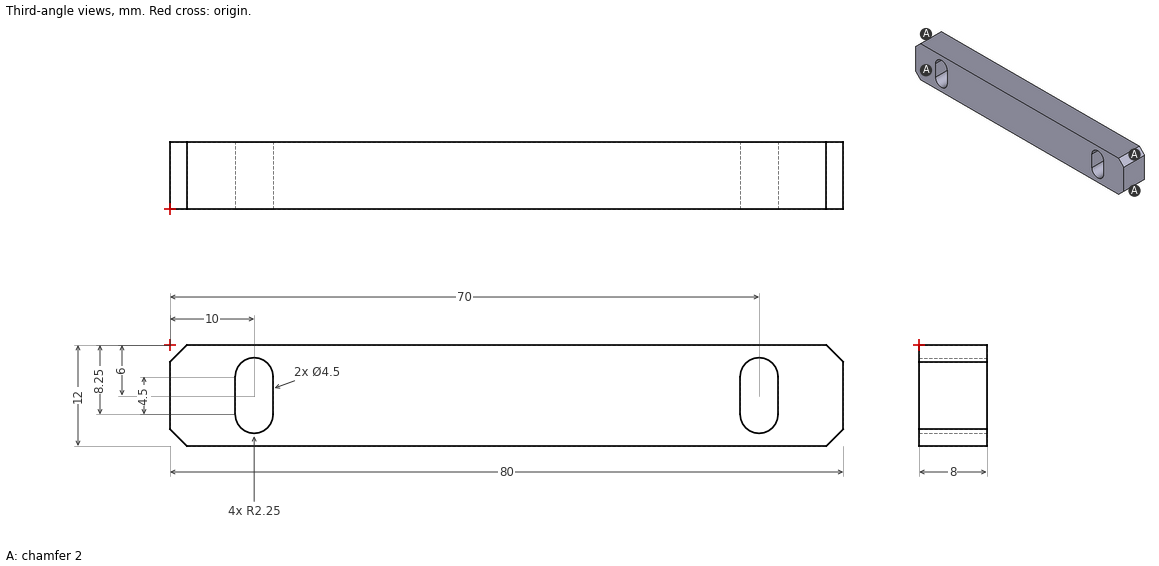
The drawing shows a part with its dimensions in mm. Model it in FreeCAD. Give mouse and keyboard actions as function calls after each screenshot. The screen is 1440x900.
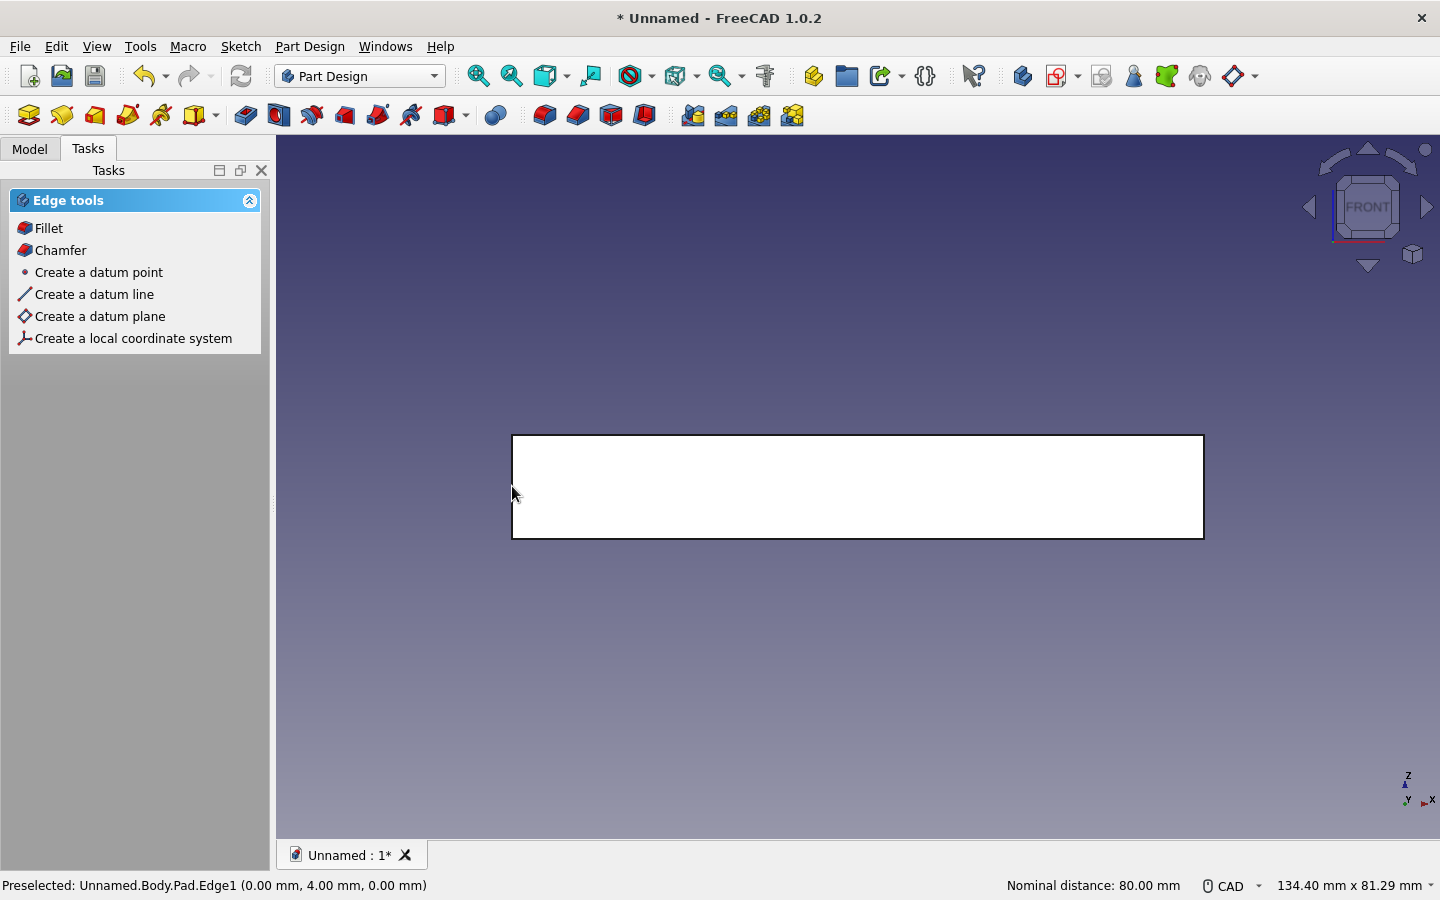
key(3)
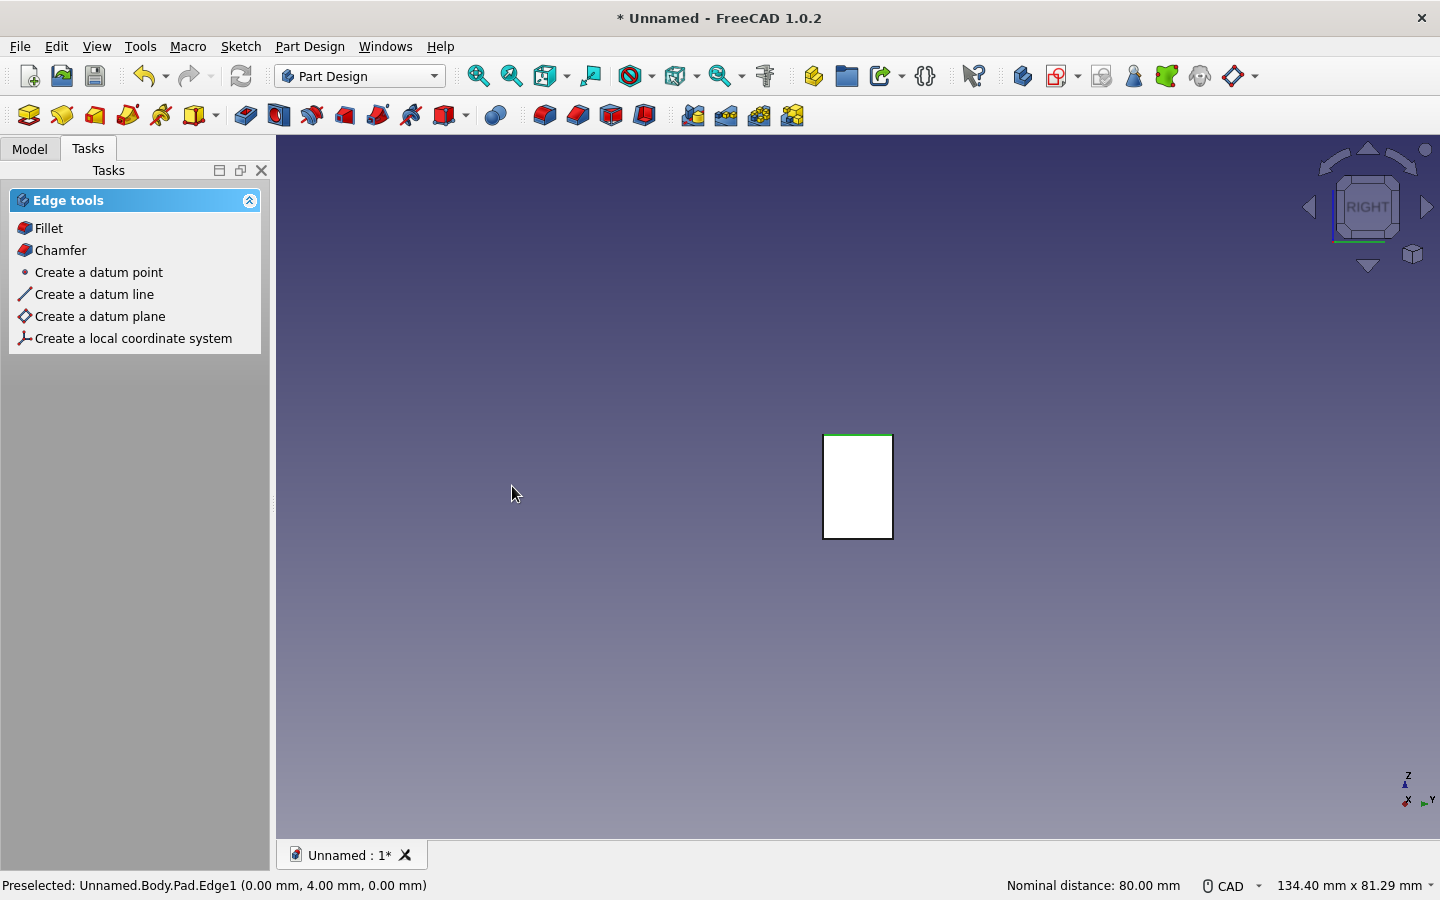
click(479, 76)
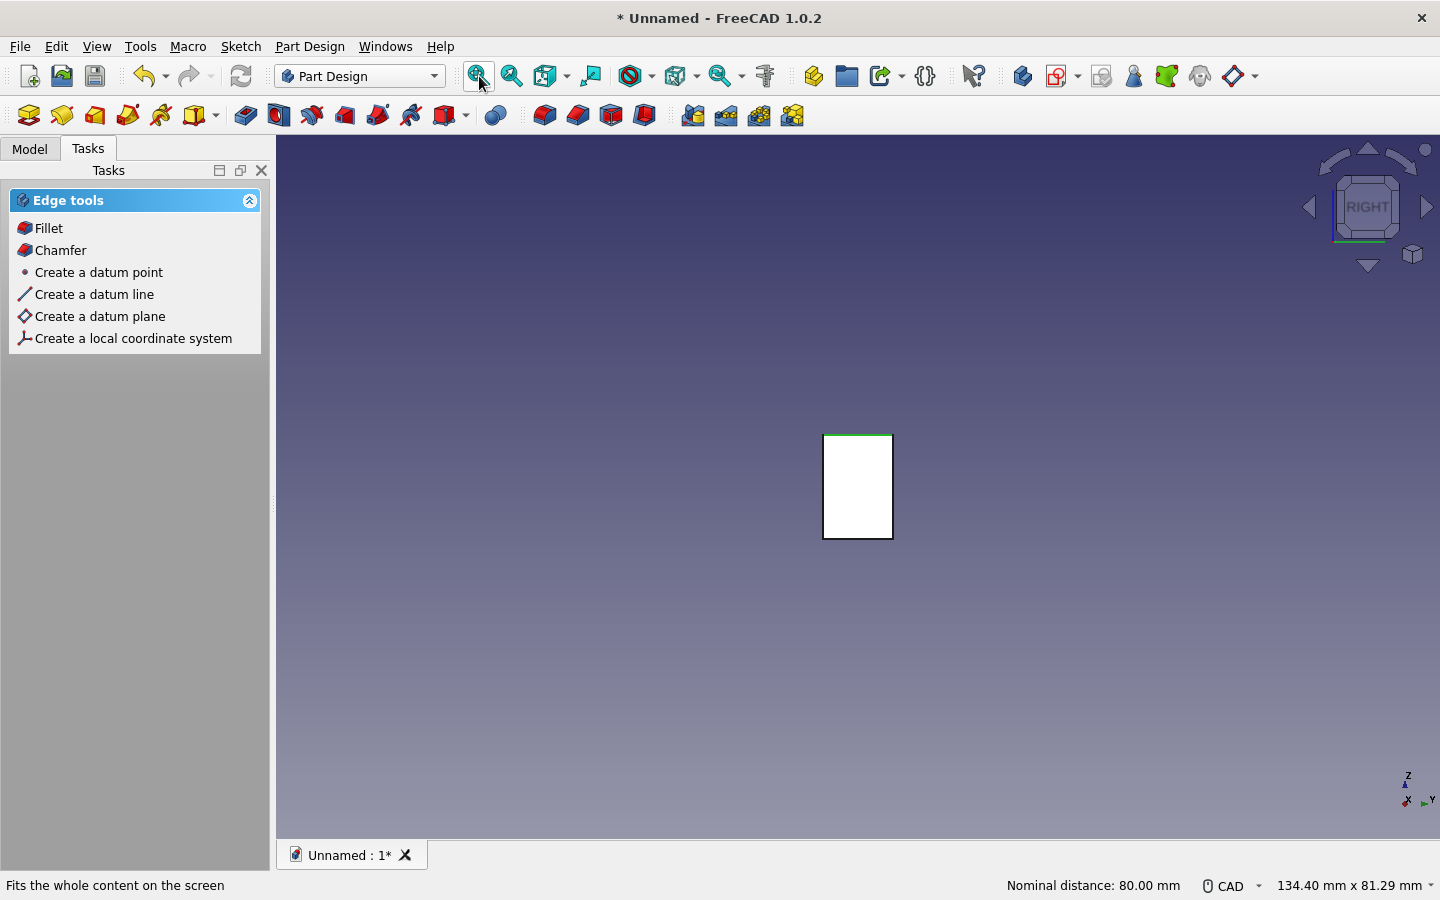
click(858, 538, ctrl)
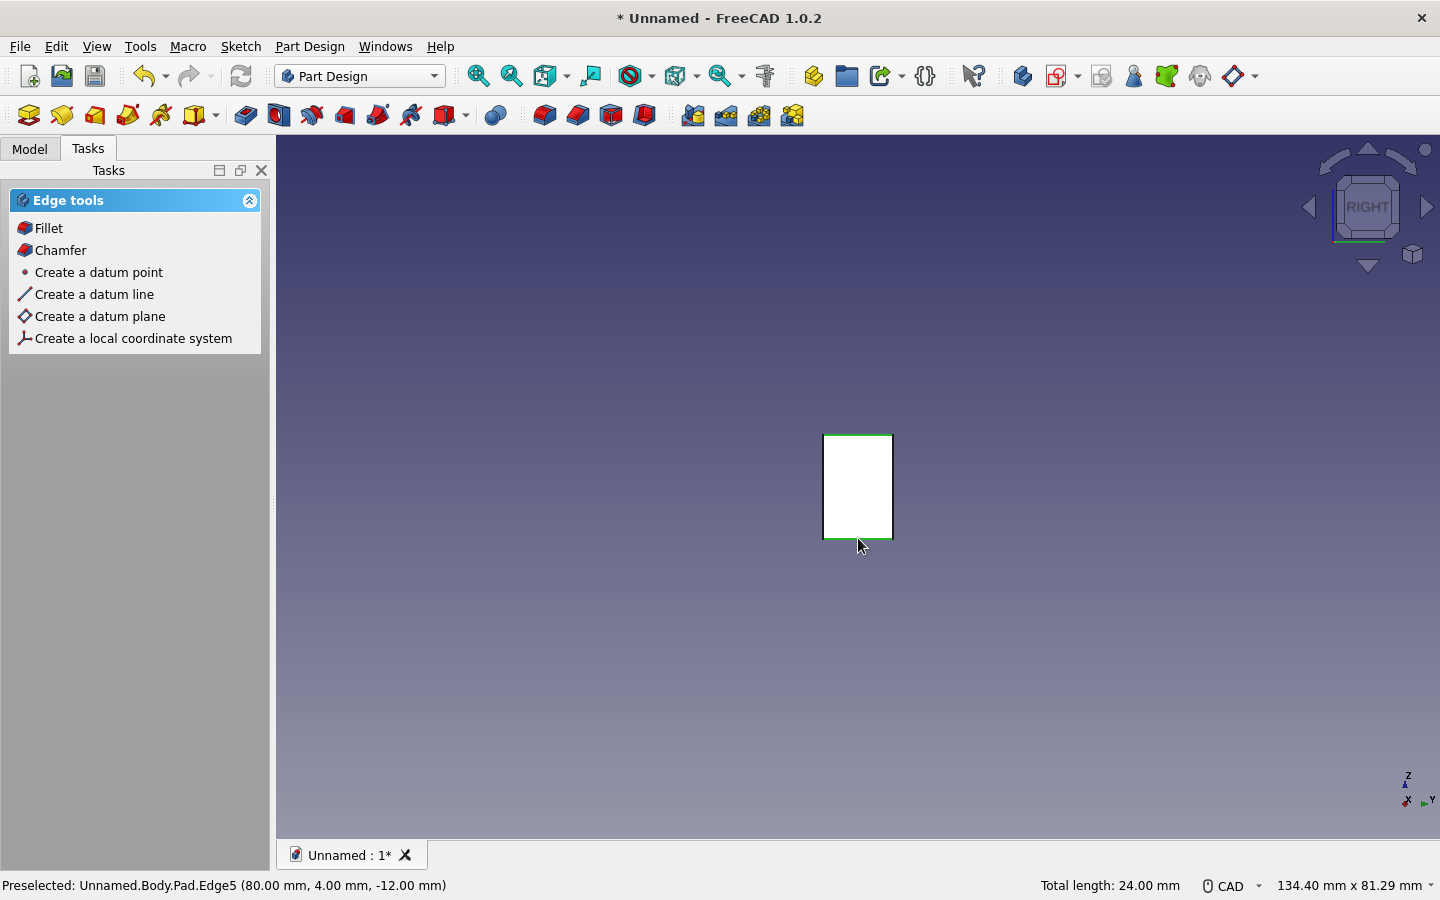
key(5)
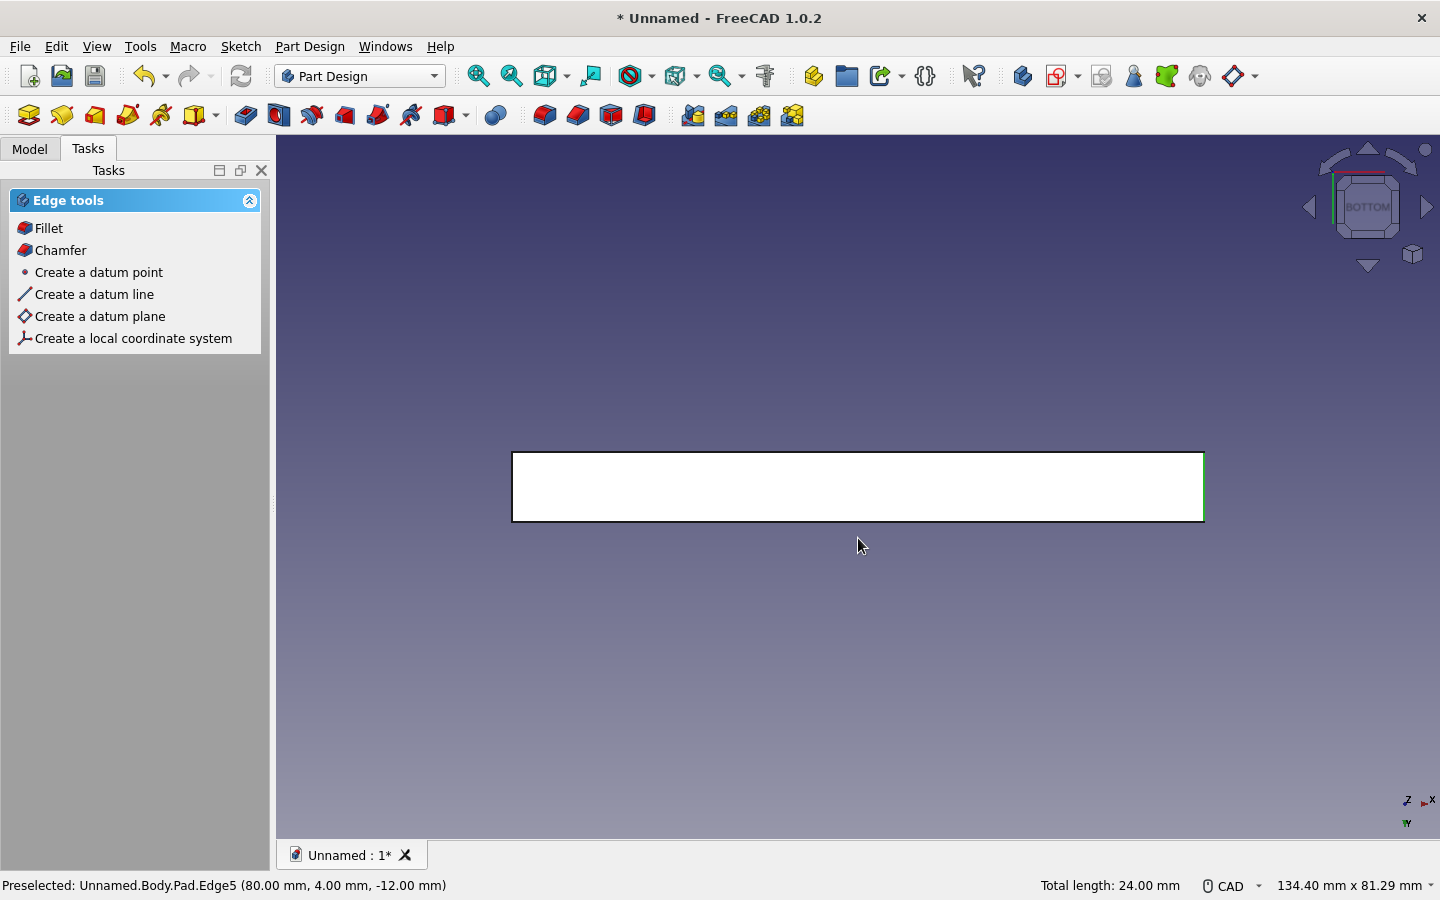
click(512, 486, ctrl)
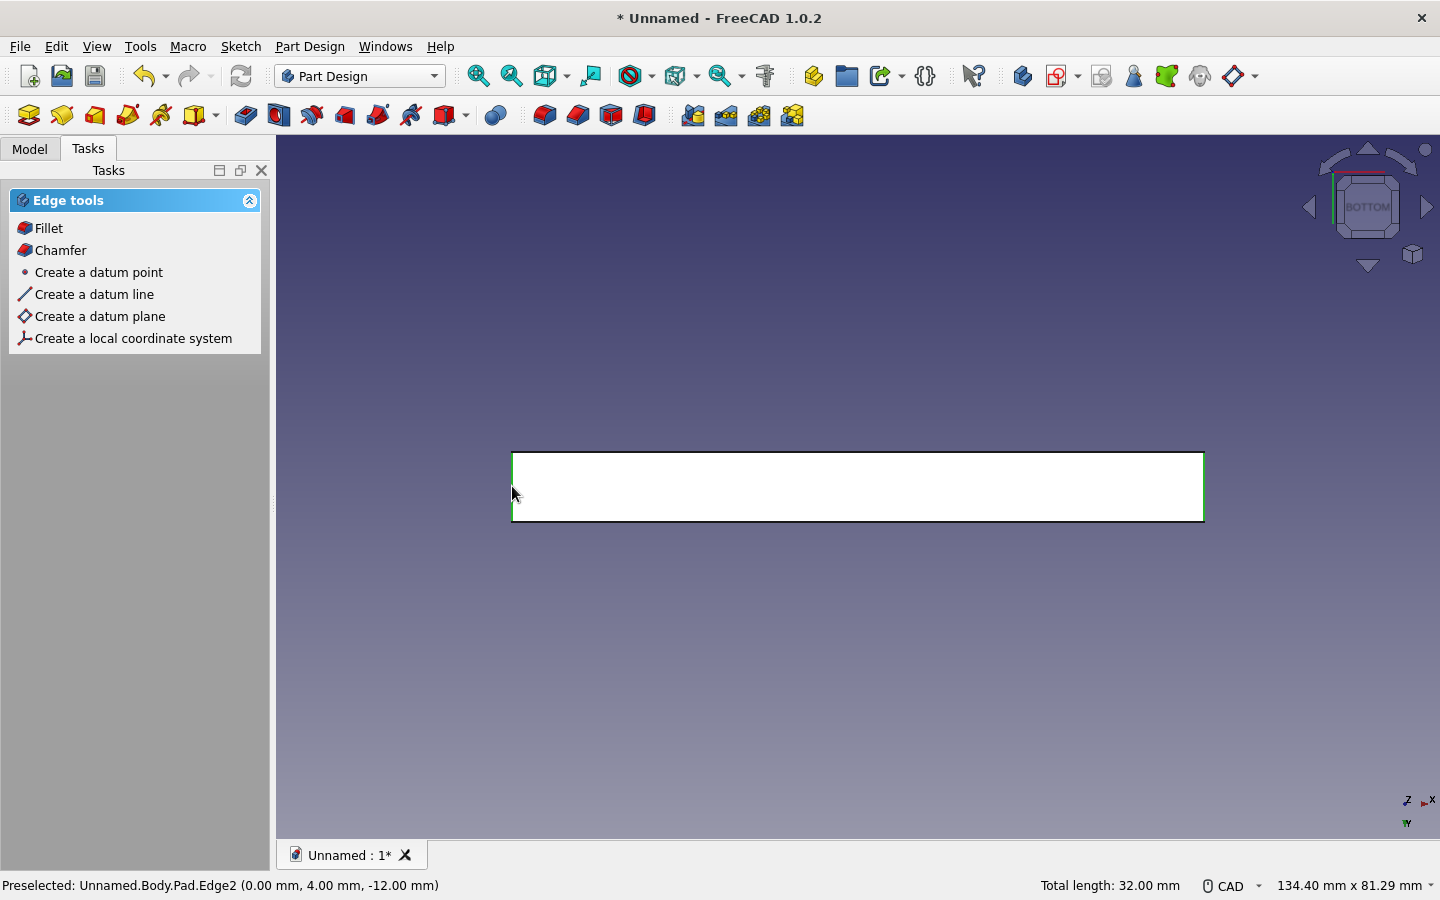
click(578, 116)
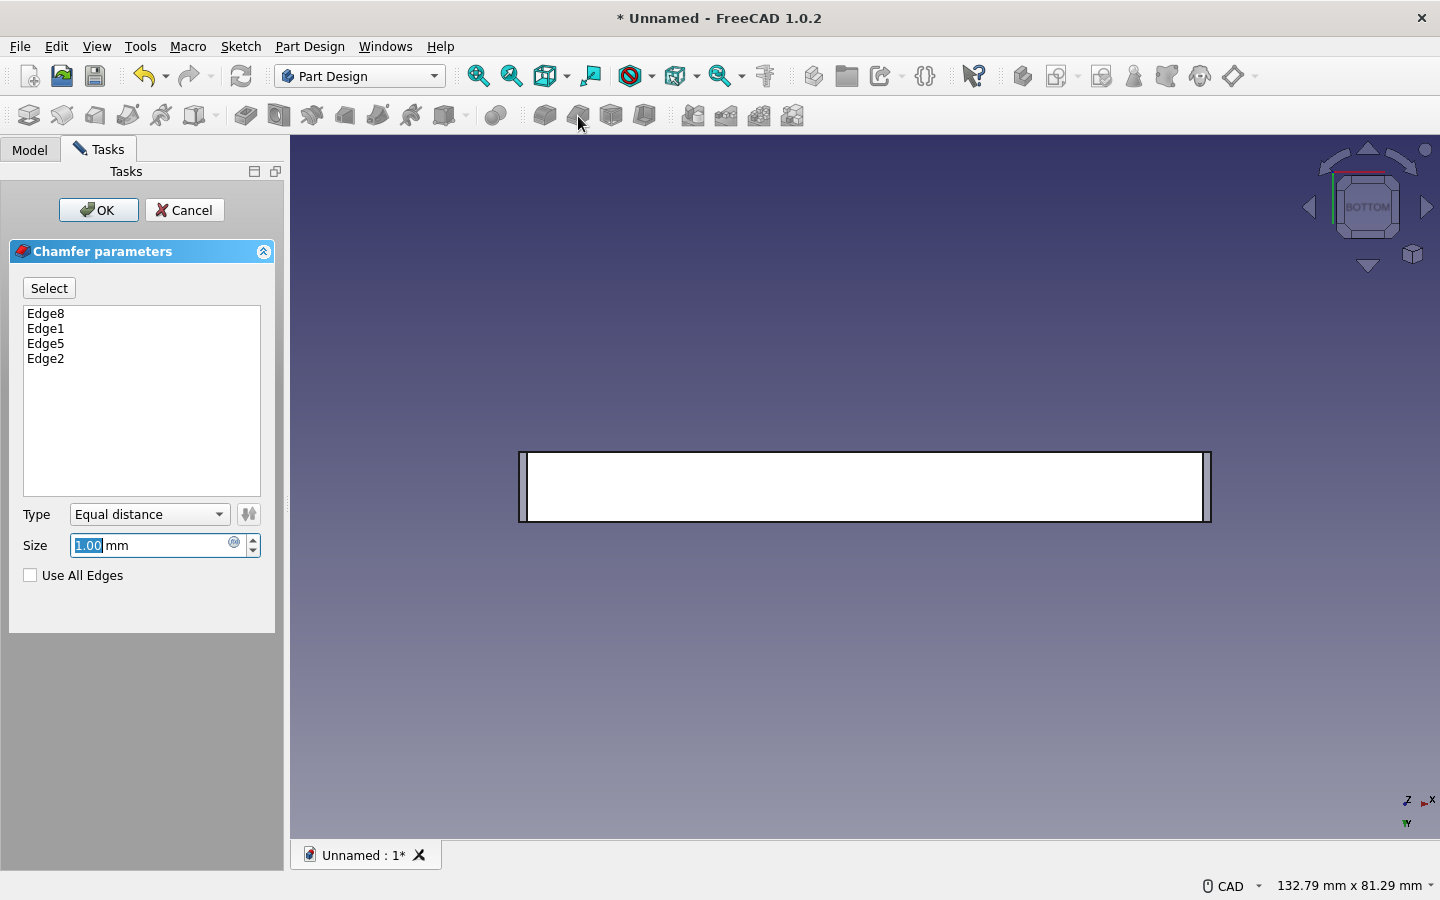
text(2)
key(Tab)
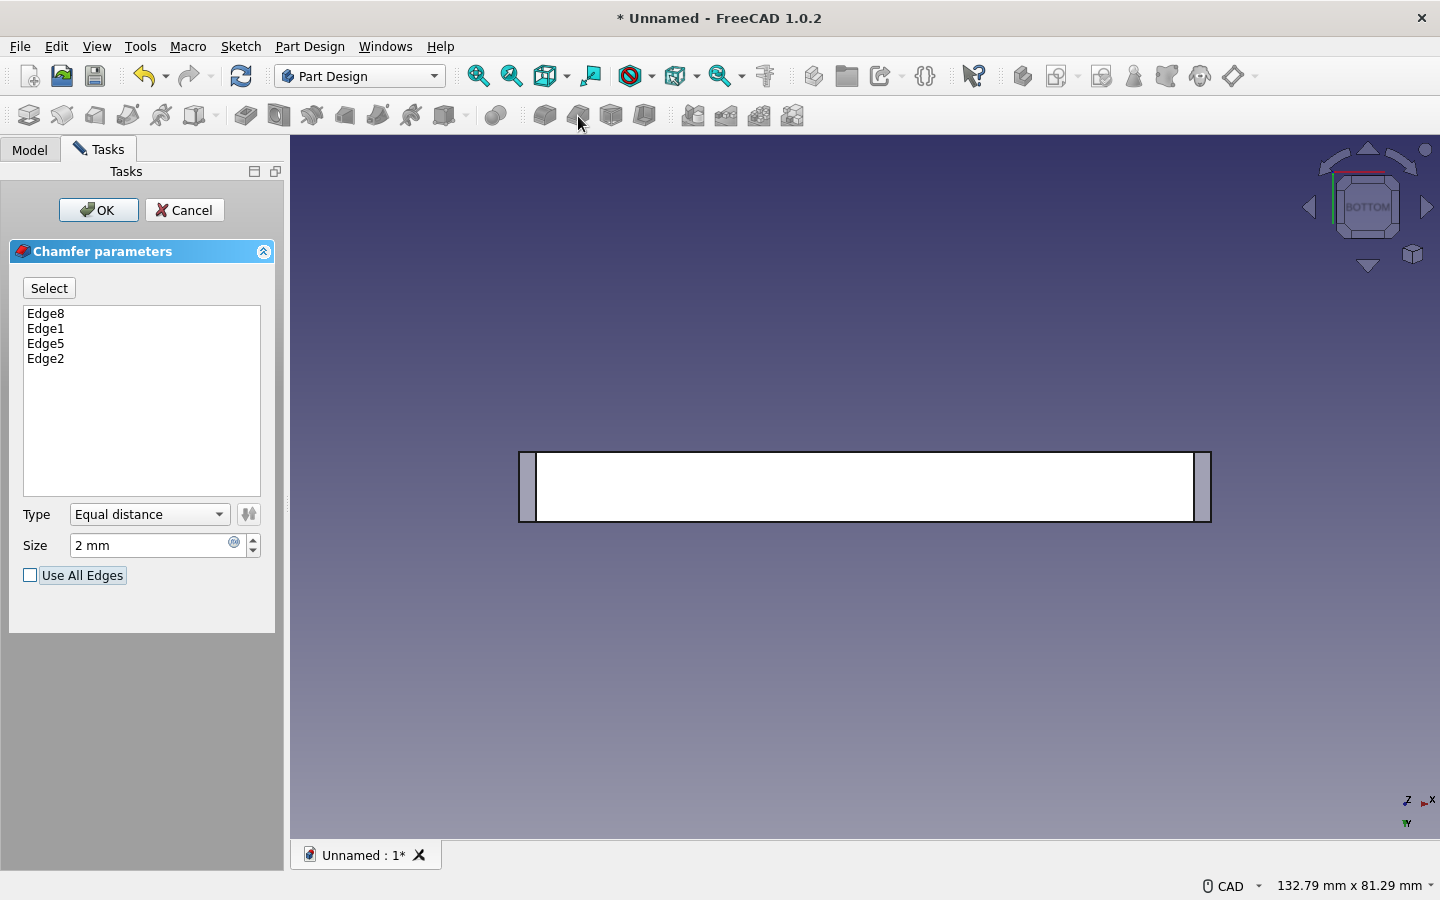
click(99, 210)